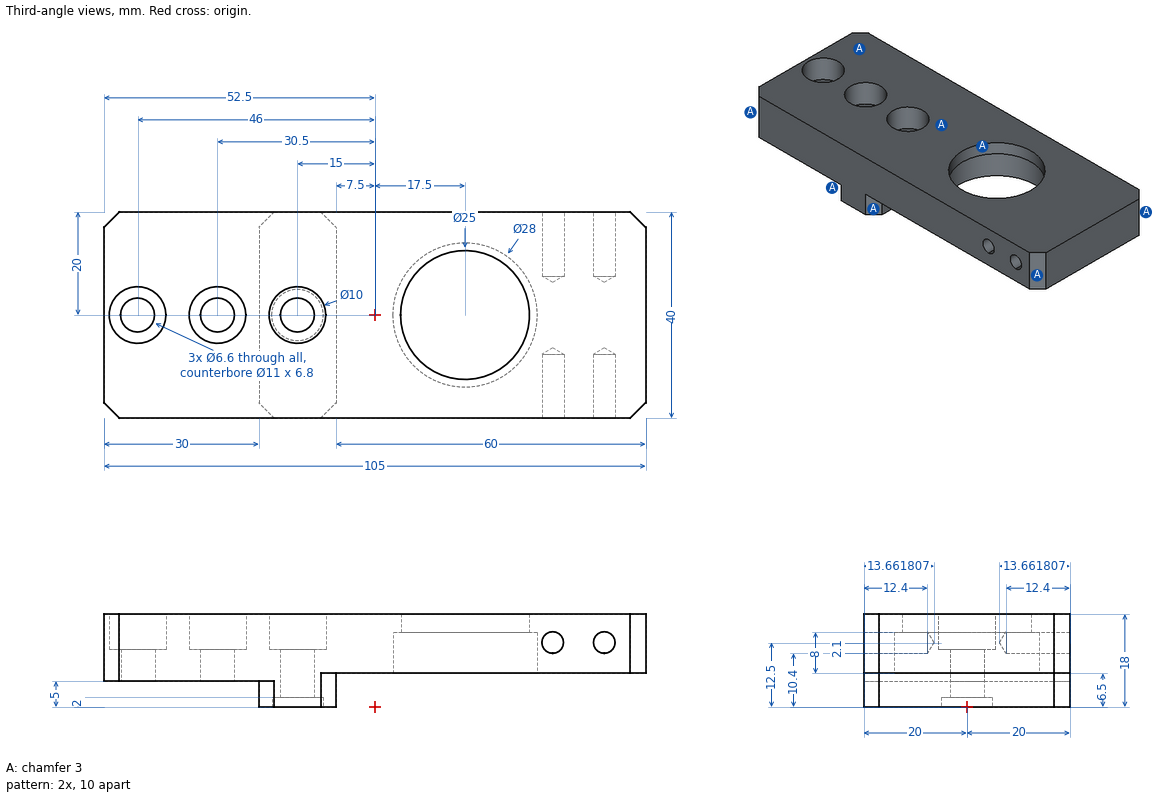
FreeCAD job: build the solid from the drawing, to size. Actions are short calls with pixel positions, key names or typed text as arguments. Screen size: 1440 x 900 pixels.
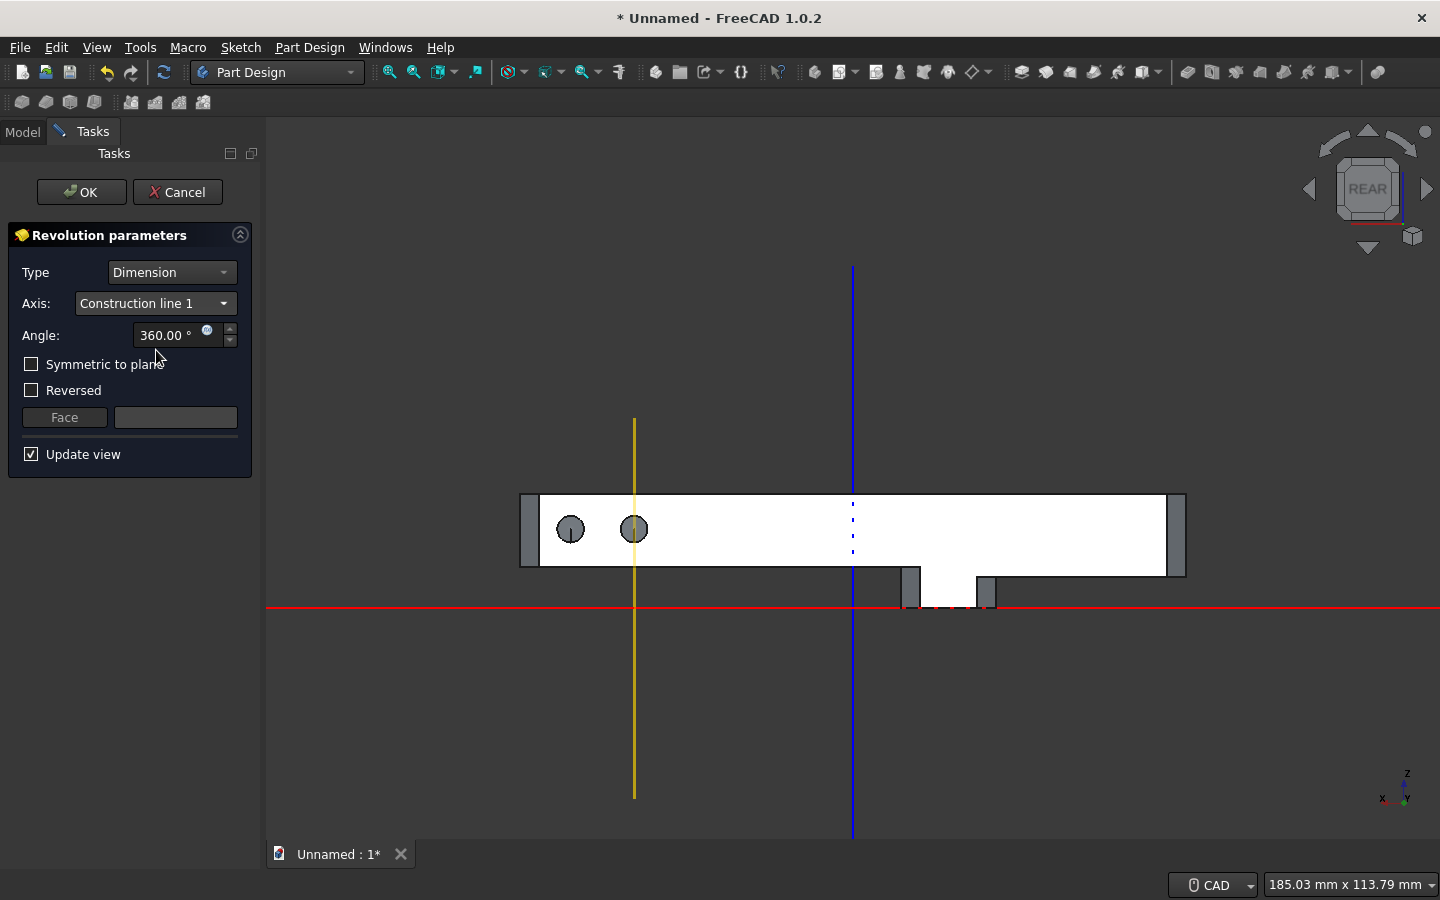
click(82, 192)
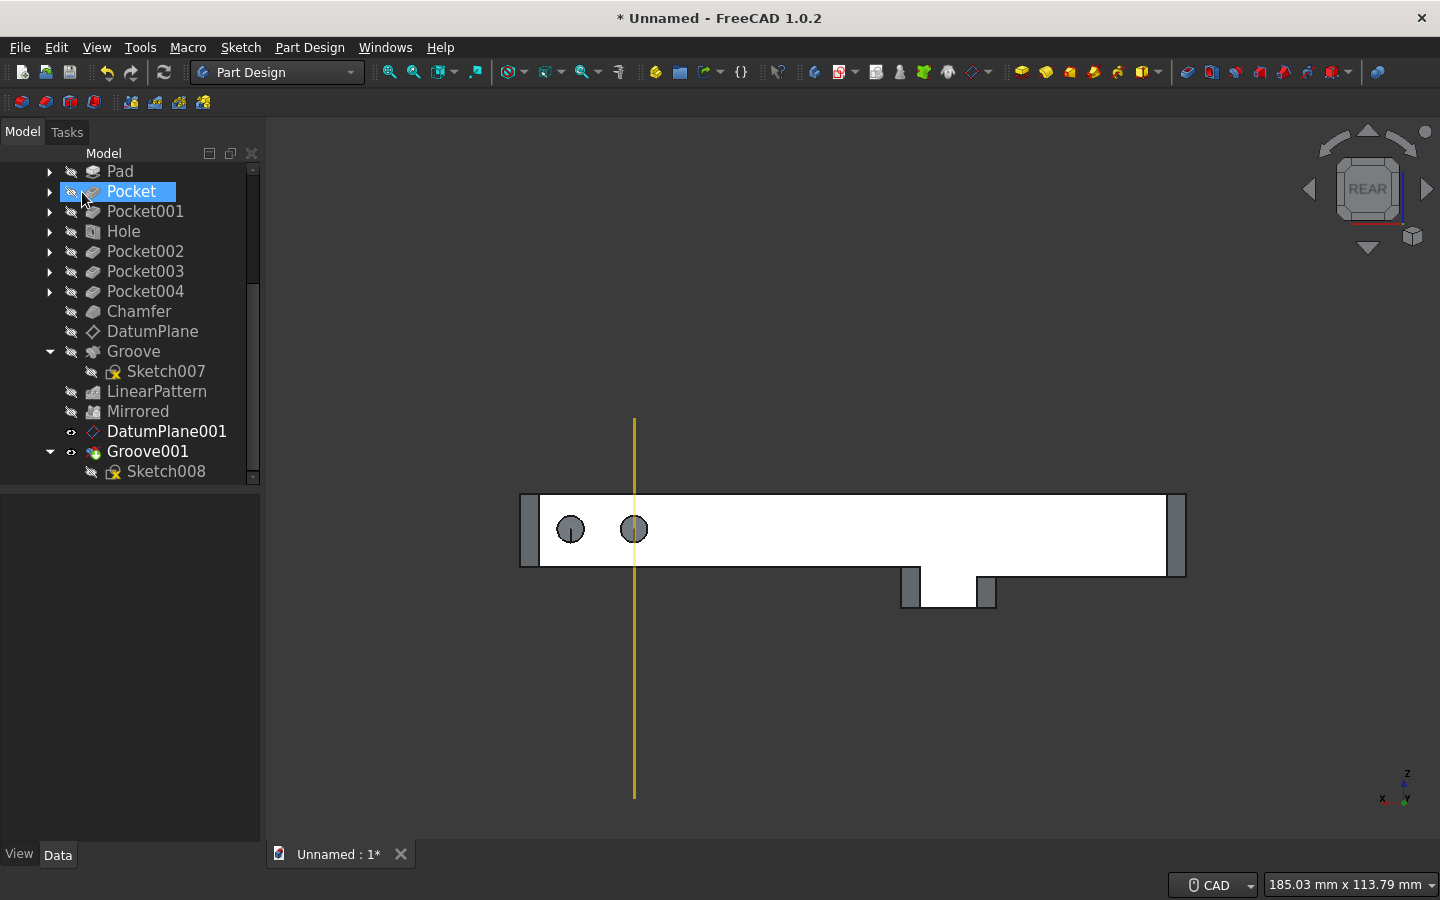
click(116, 432)
key(space)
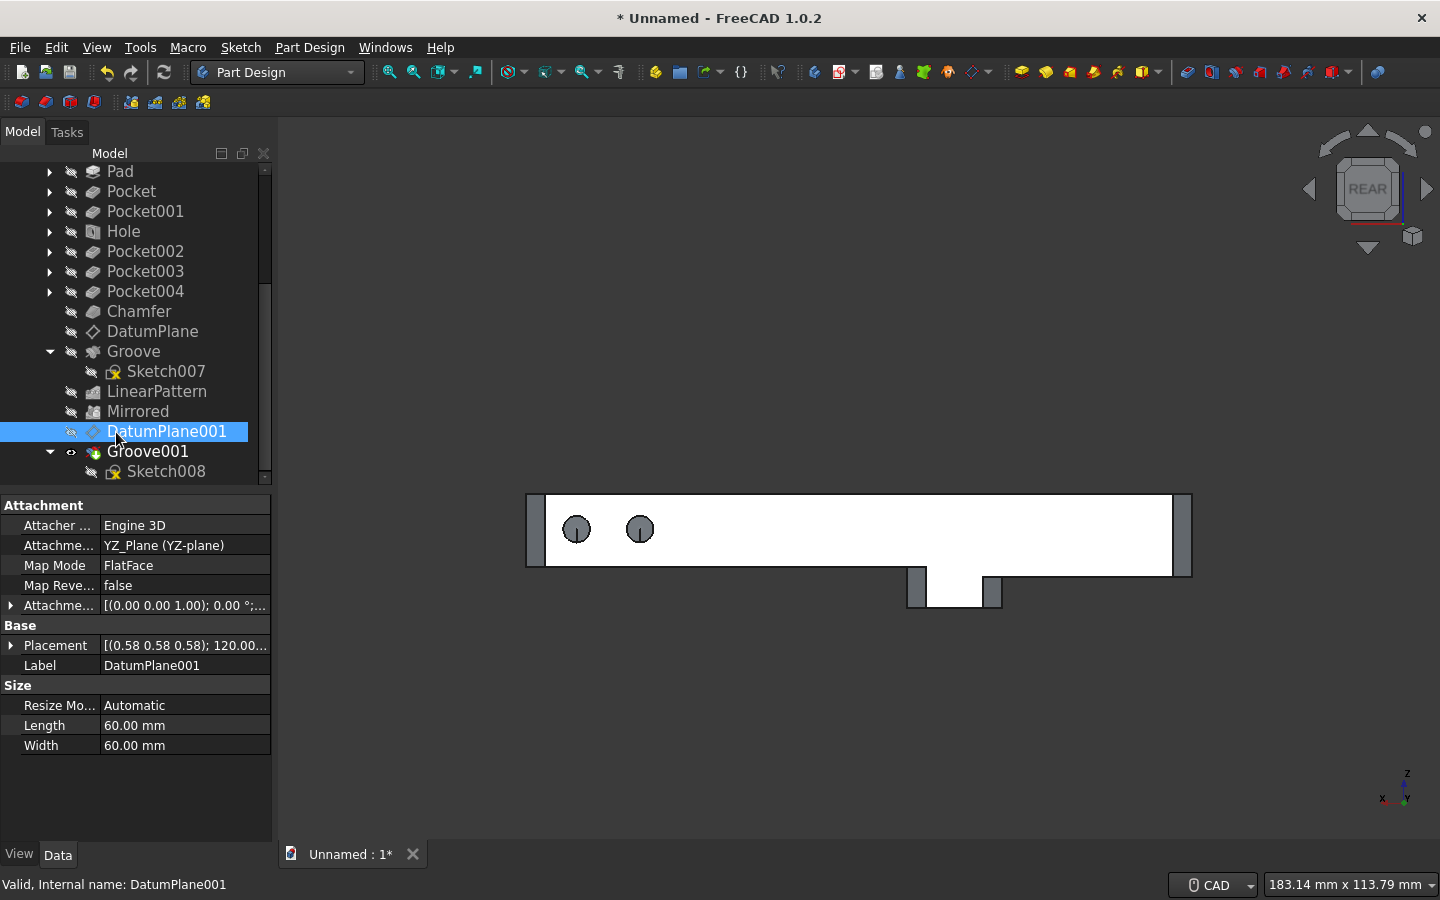
key(0)